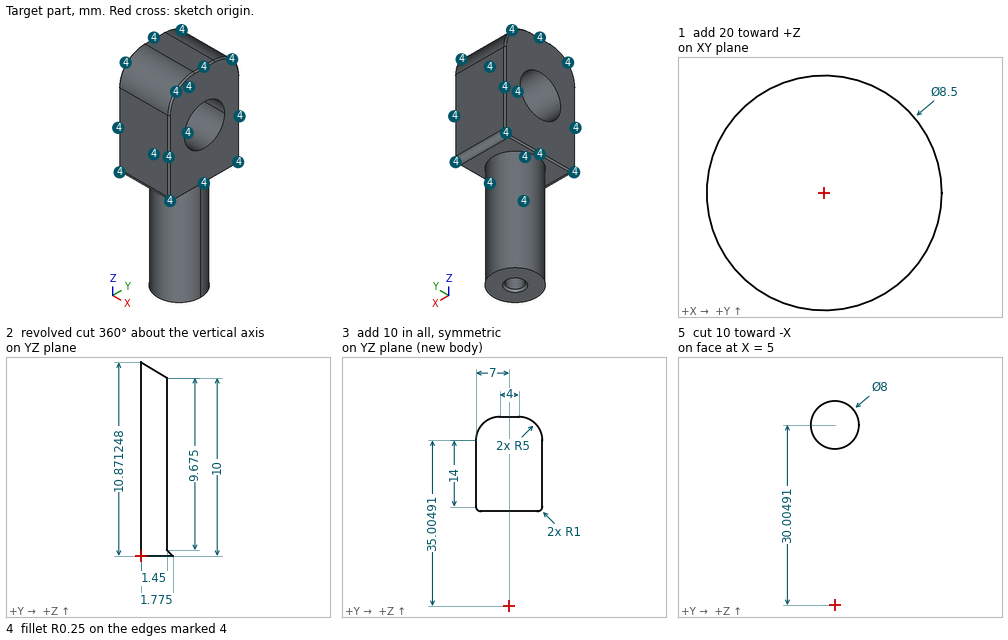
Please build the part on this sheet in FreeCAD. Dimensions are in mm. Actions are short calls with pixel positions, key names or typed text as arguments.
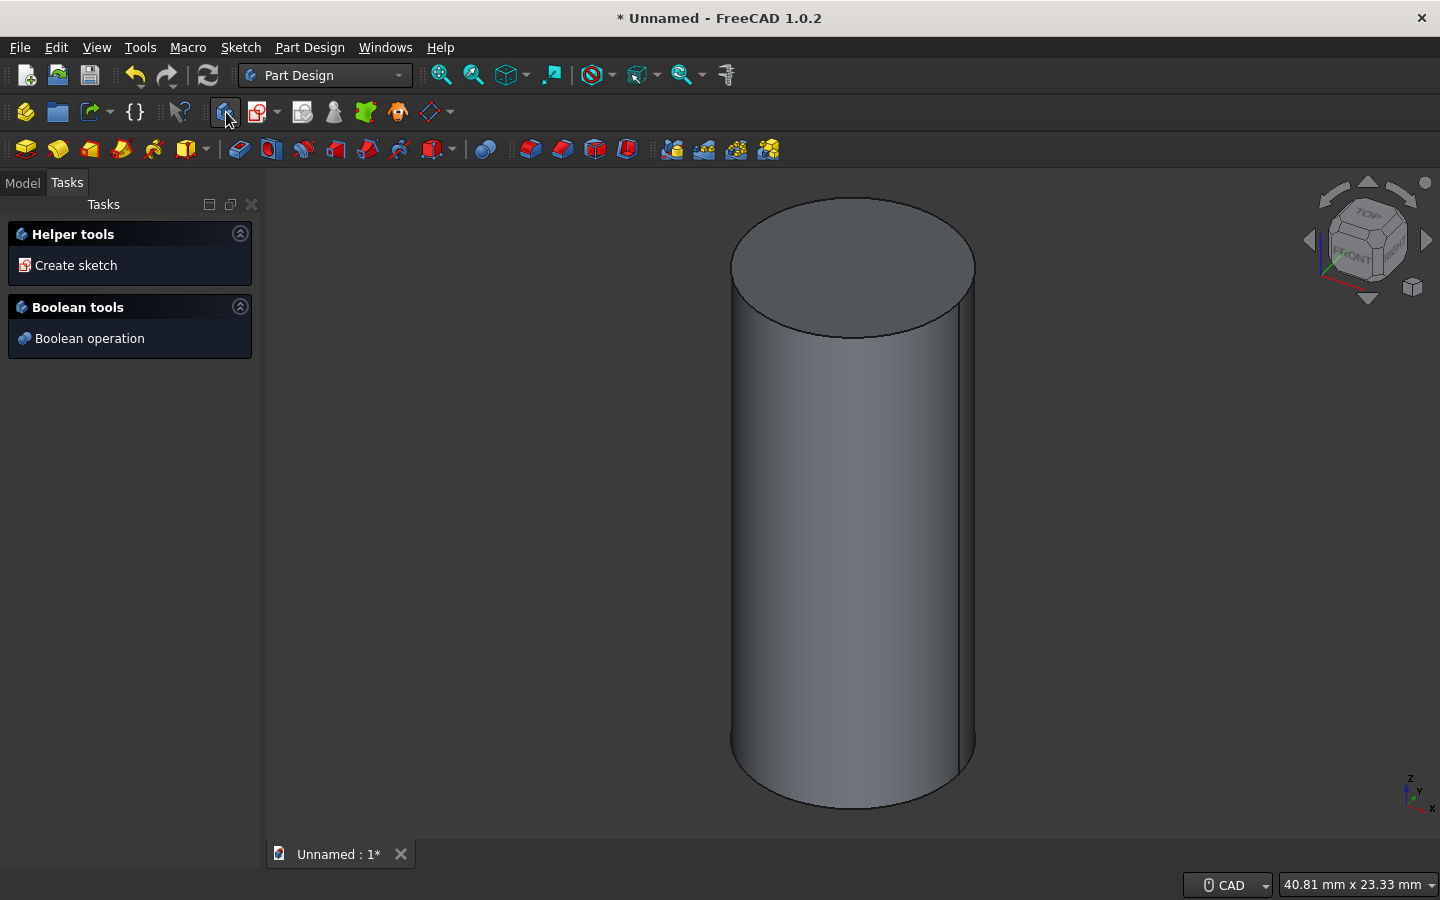
click(306, 799)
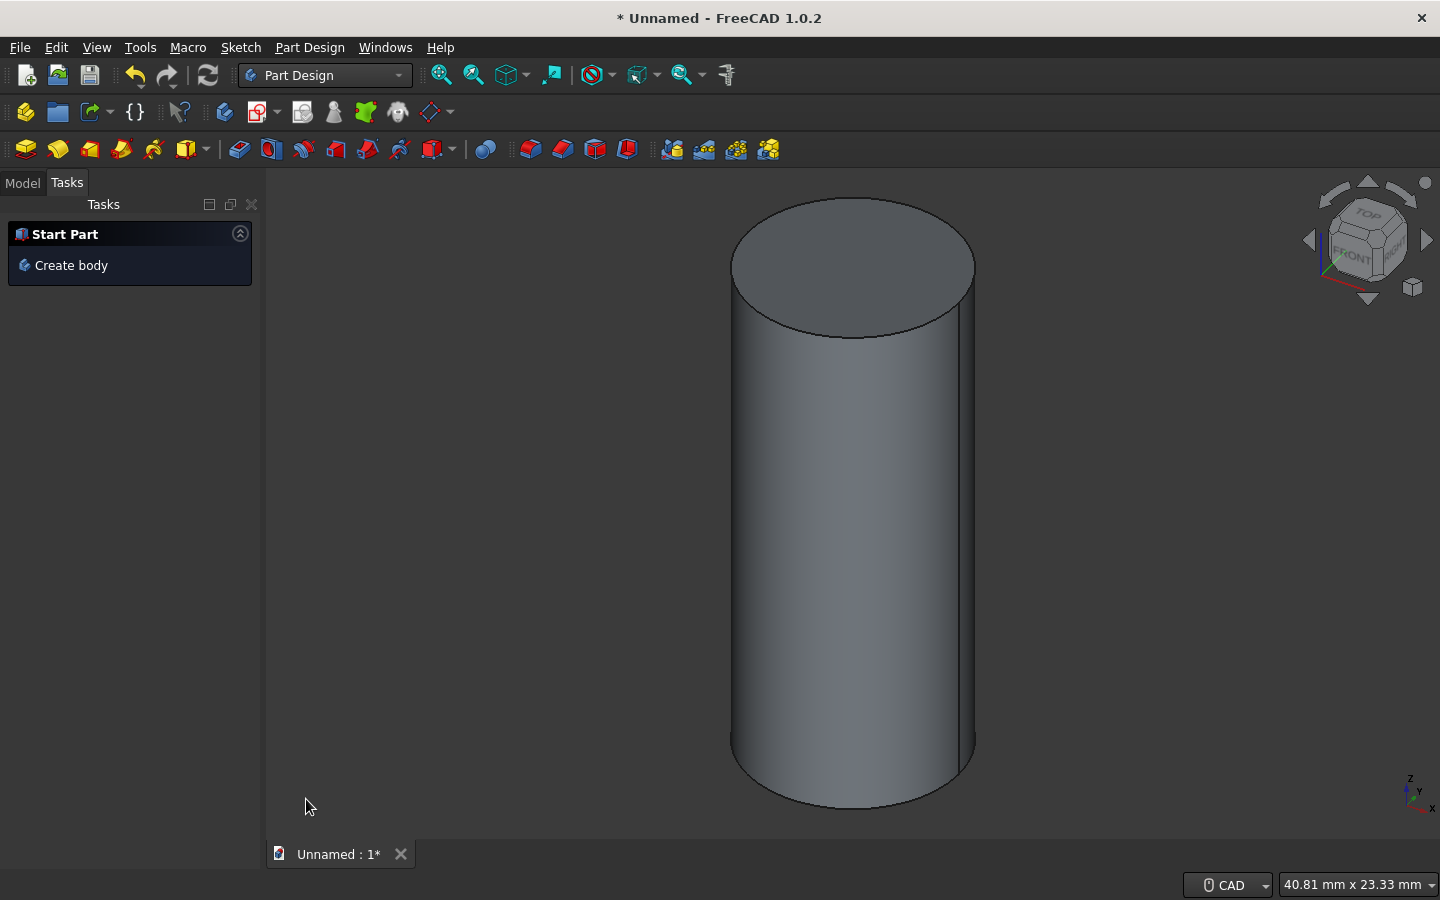
click(258, 112)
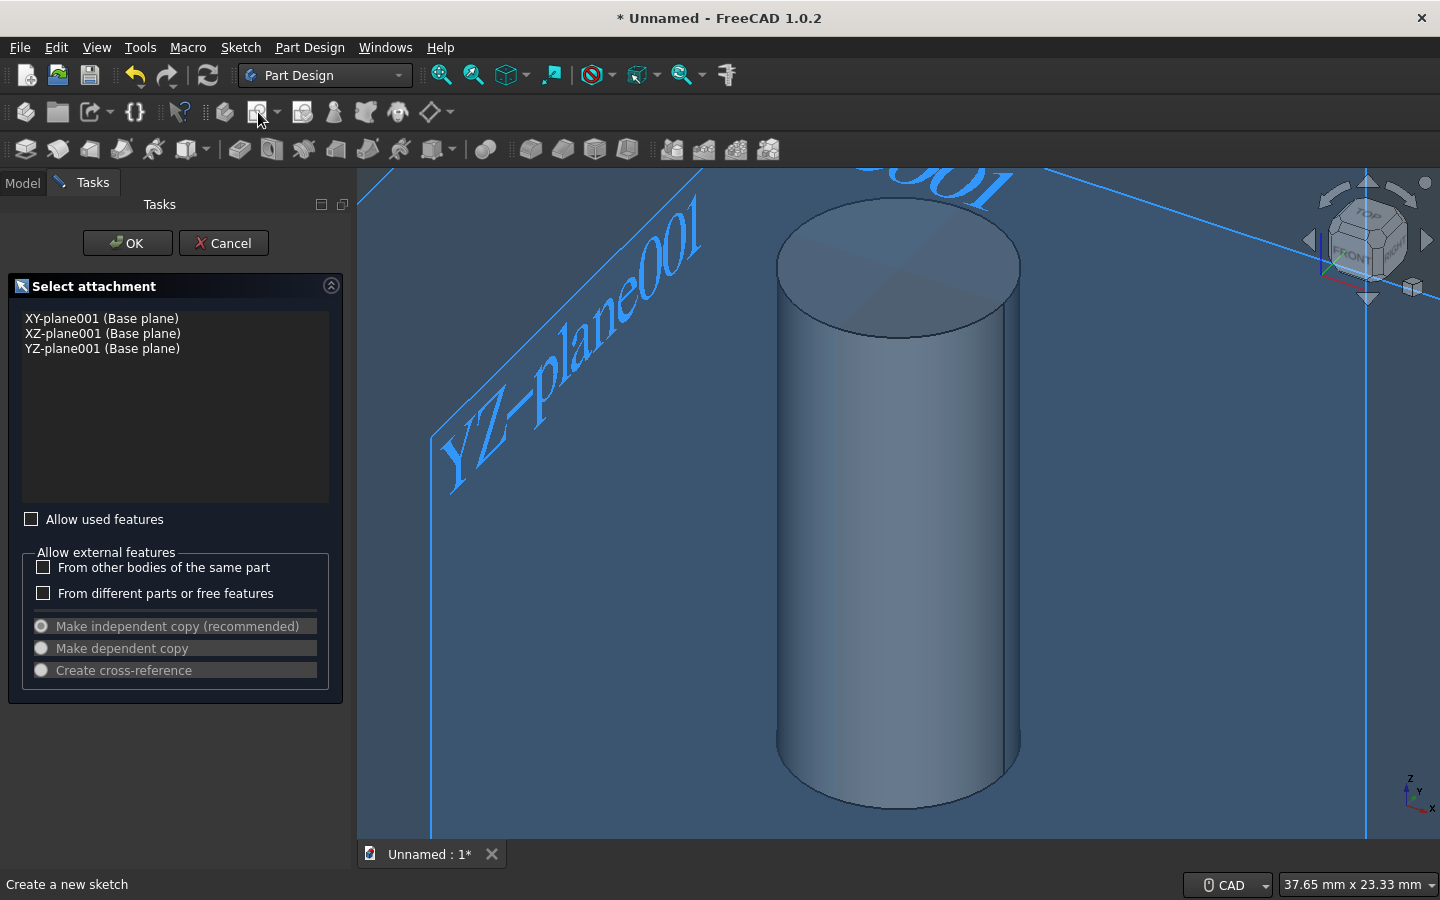
click(82, 348)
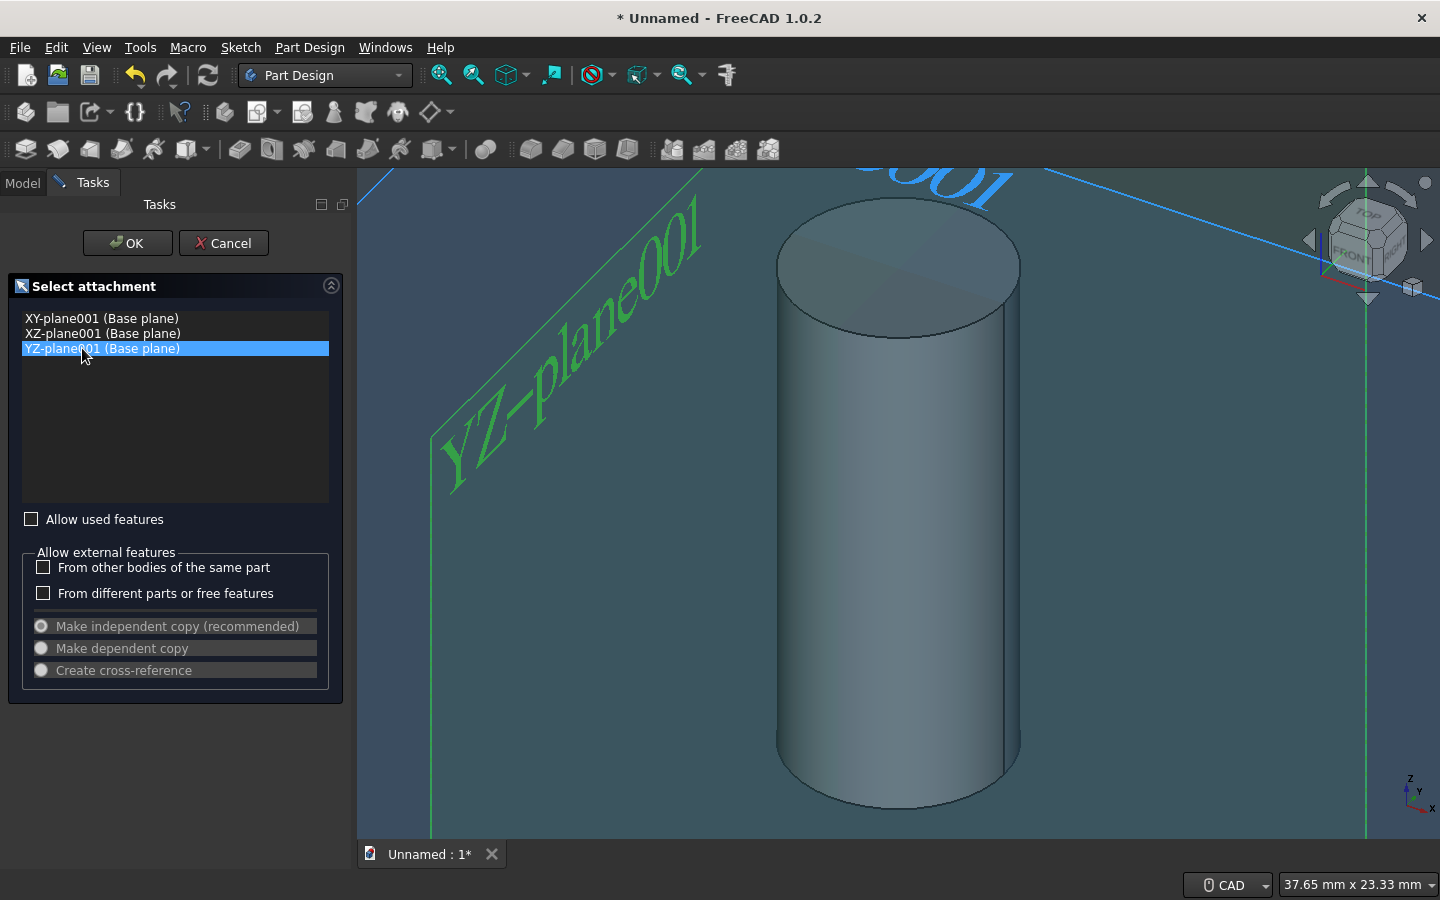
click(128, 243)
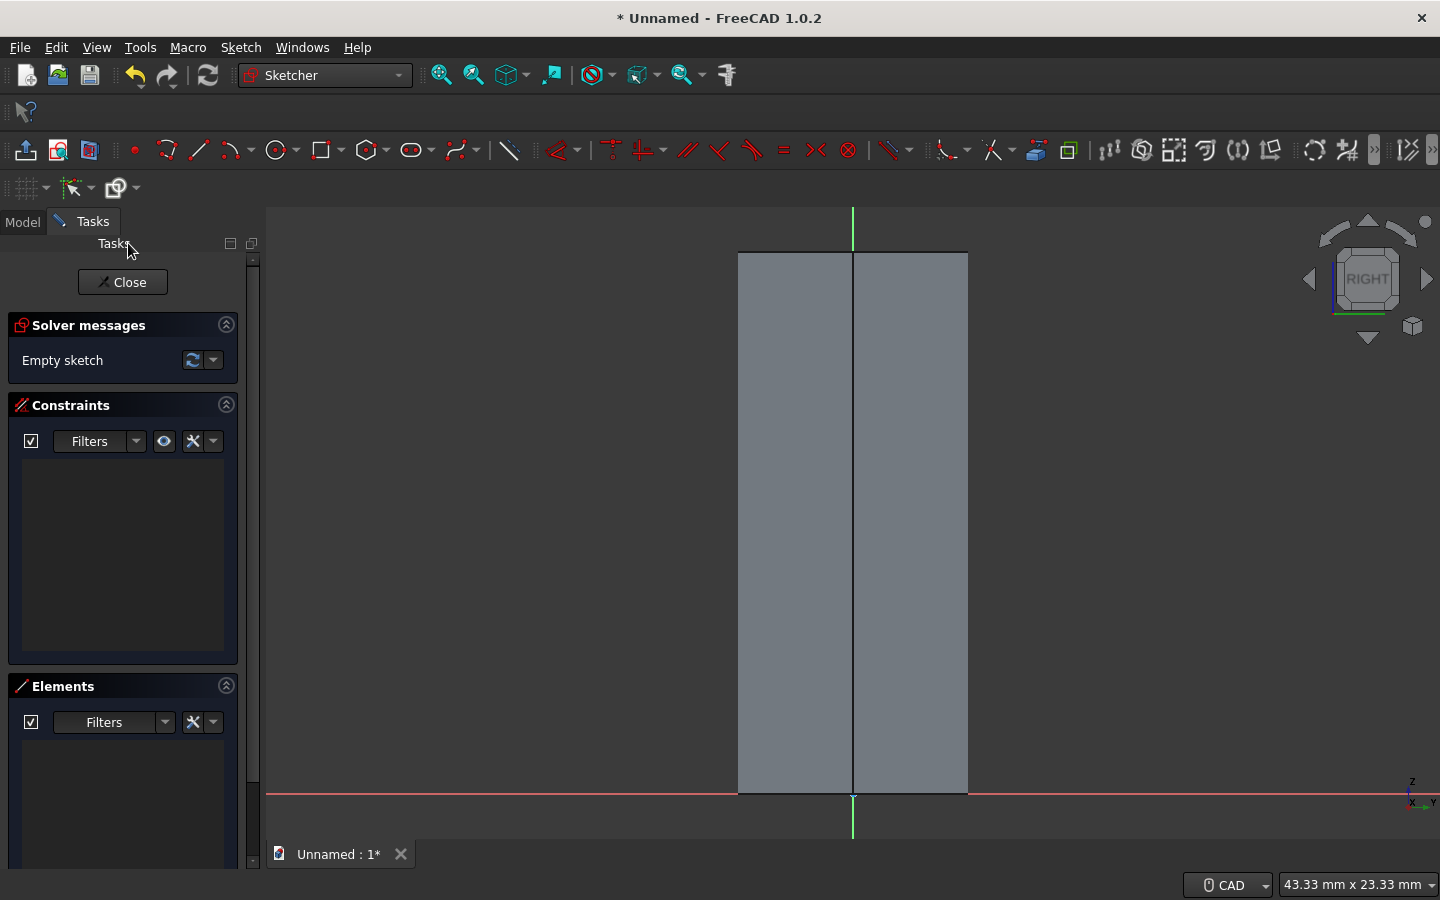
scroll(745, 681, down, 5)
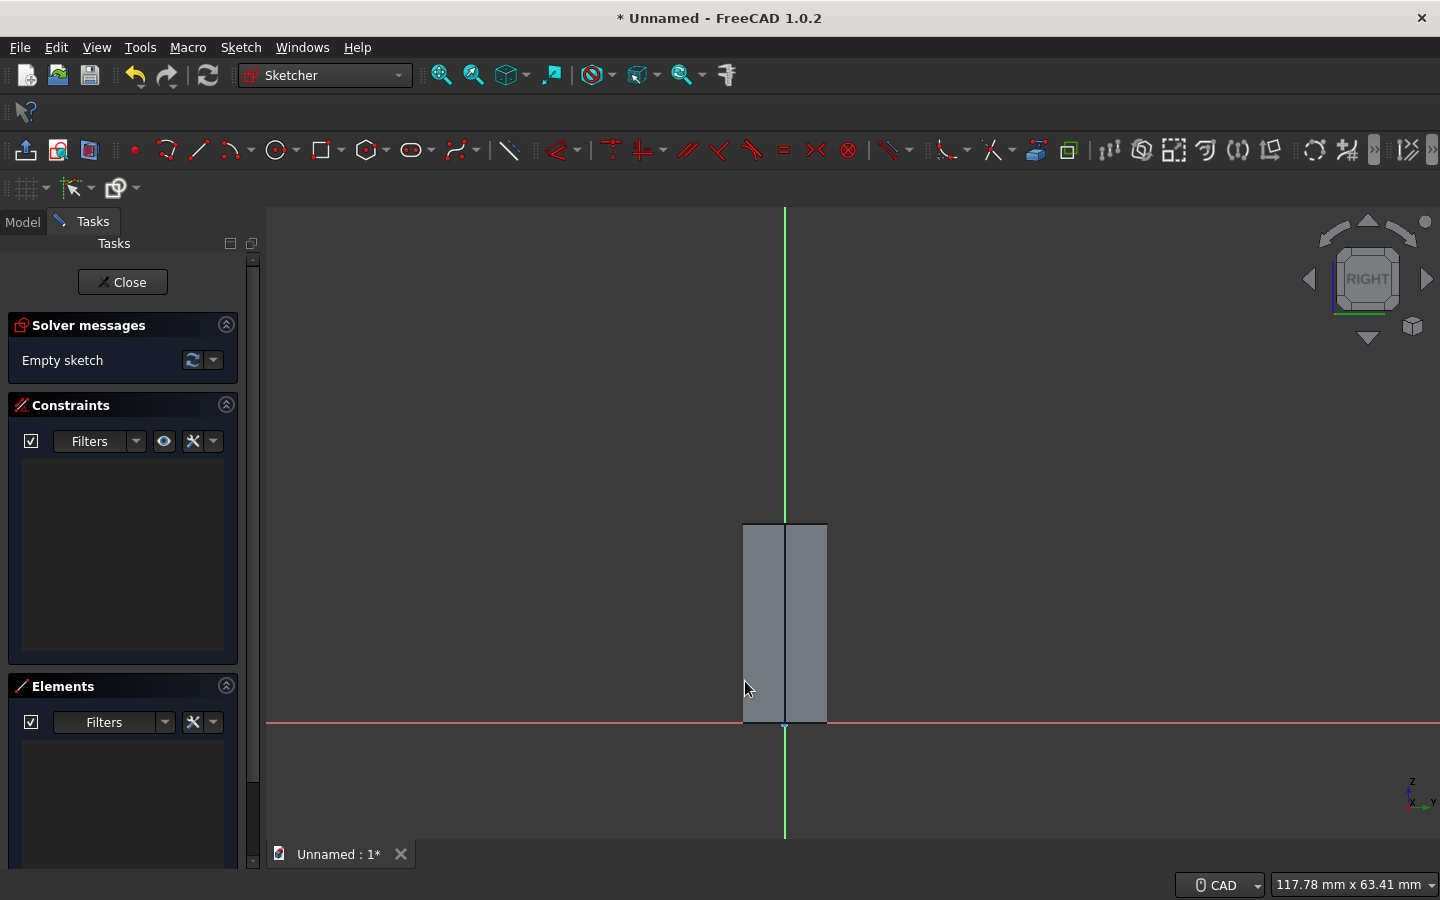
click(200, 150)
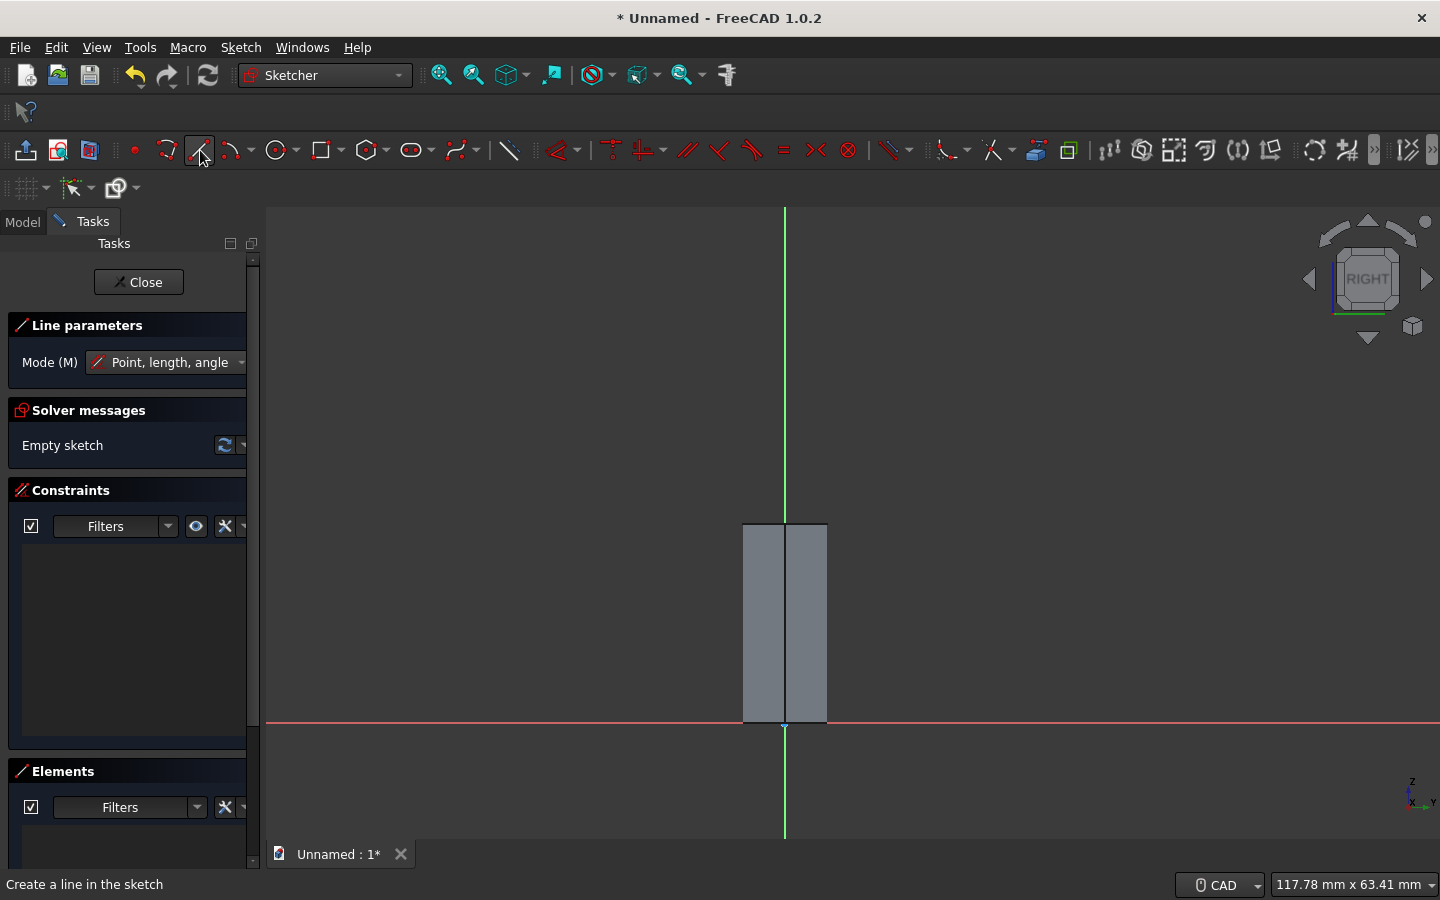
click(715, 374)
click(715, 514)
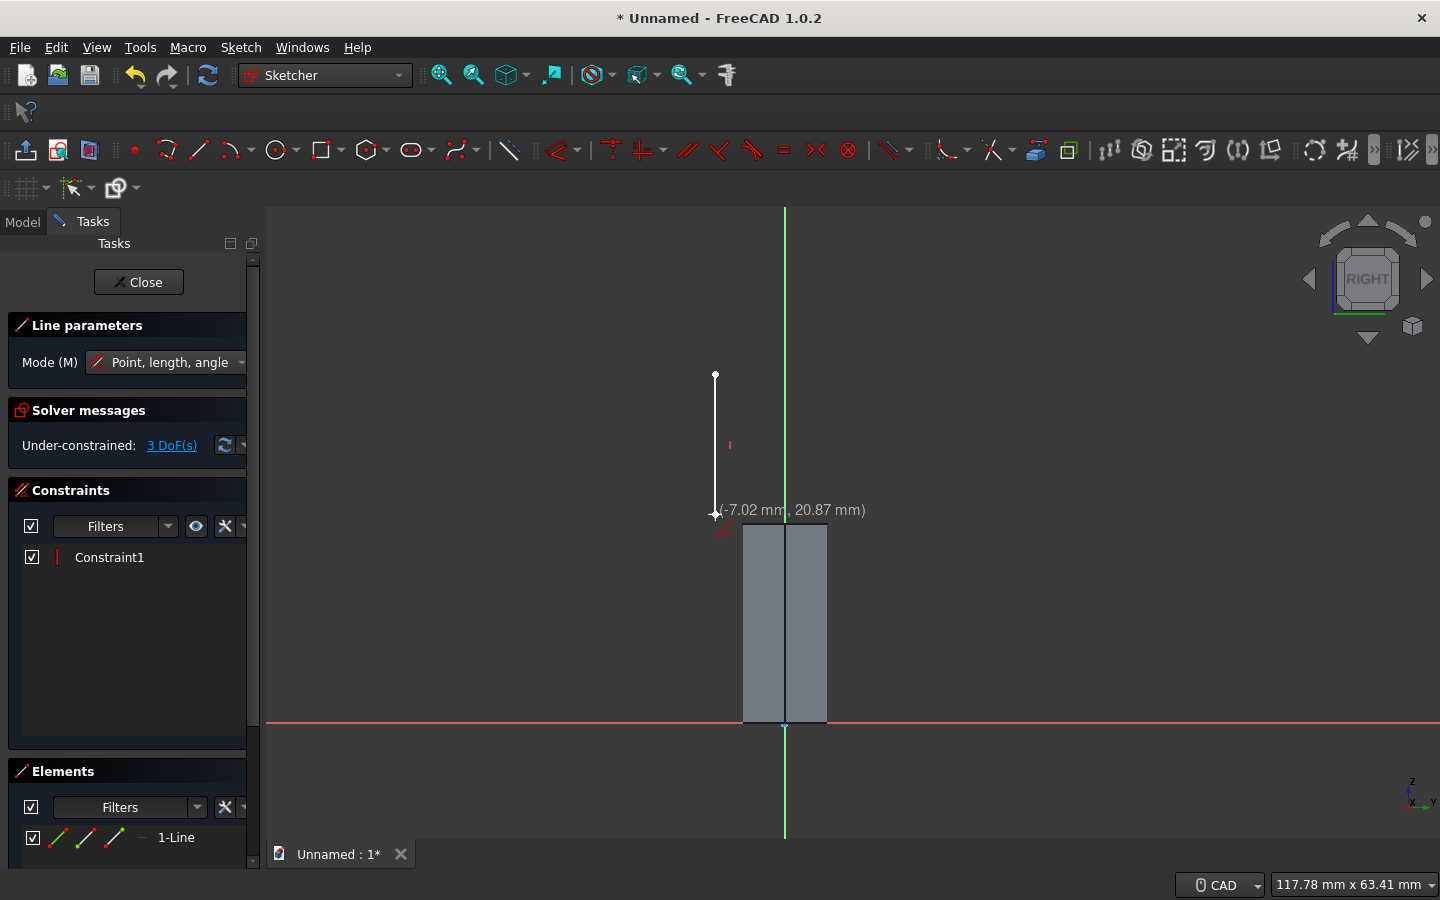
click(725, 524)
click(845, 524)